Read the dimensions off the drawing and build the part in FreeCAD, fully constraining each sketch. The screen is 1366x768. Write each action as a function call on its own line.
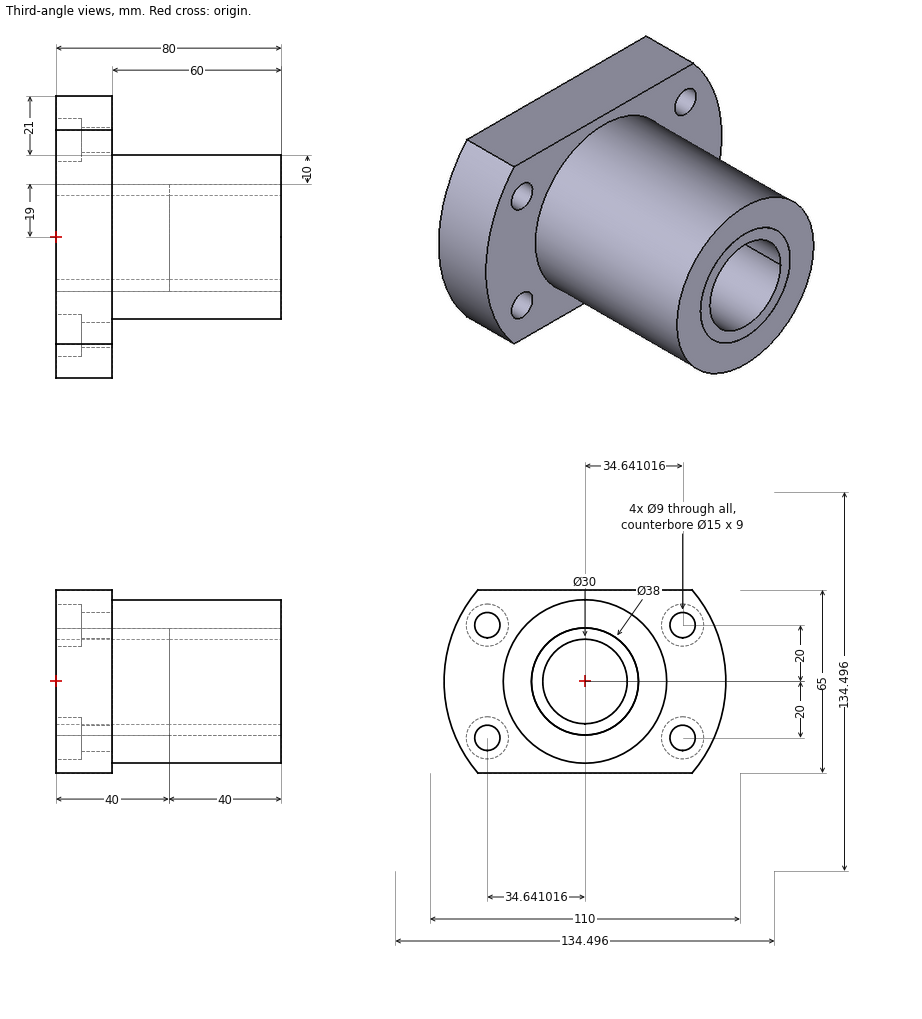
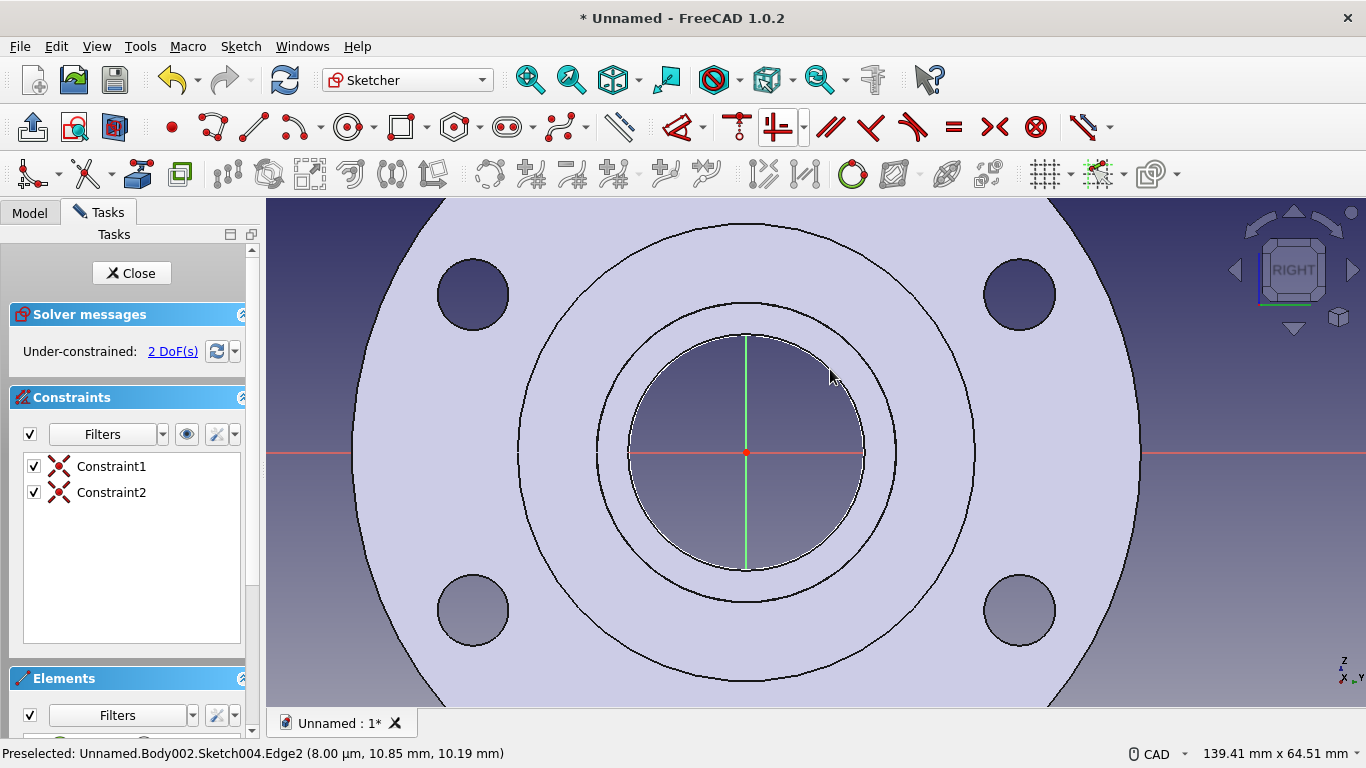
key(d)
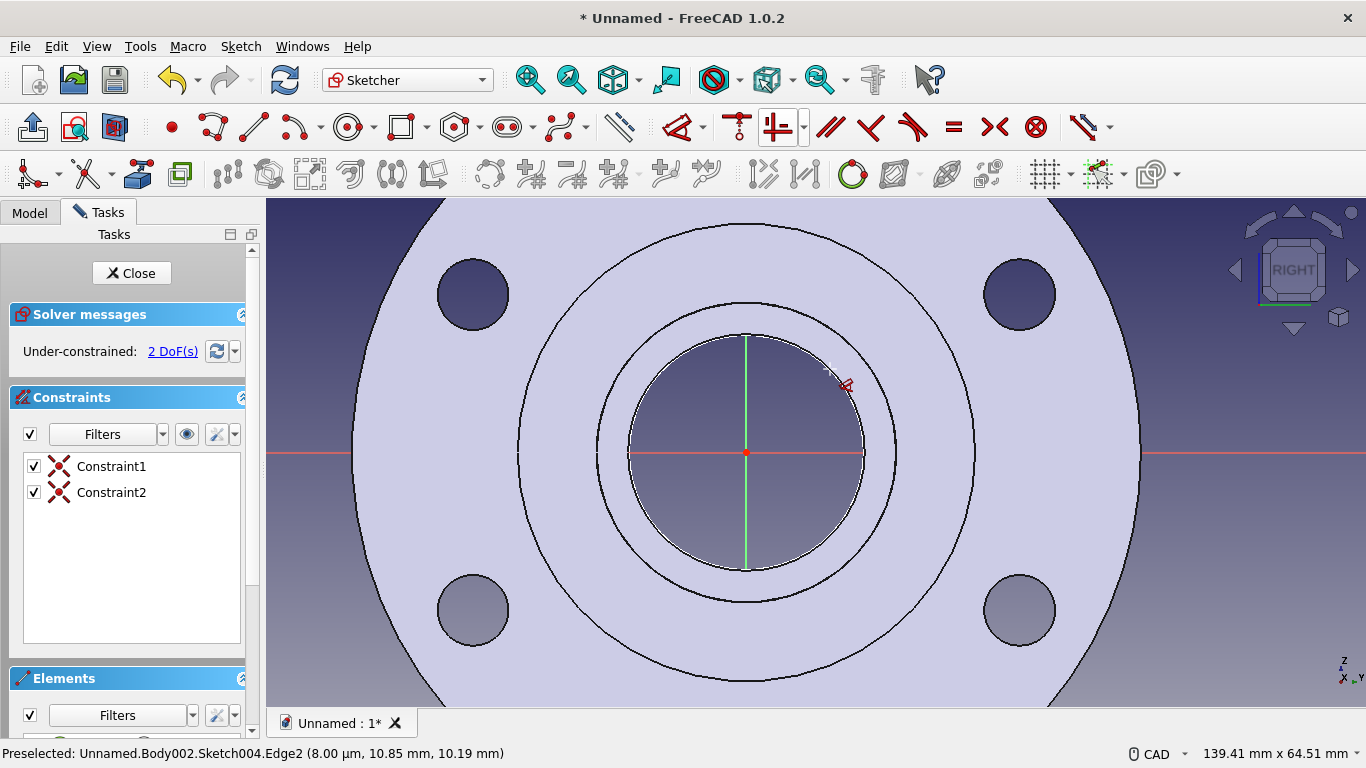
click(852, 347)
click(875, 324)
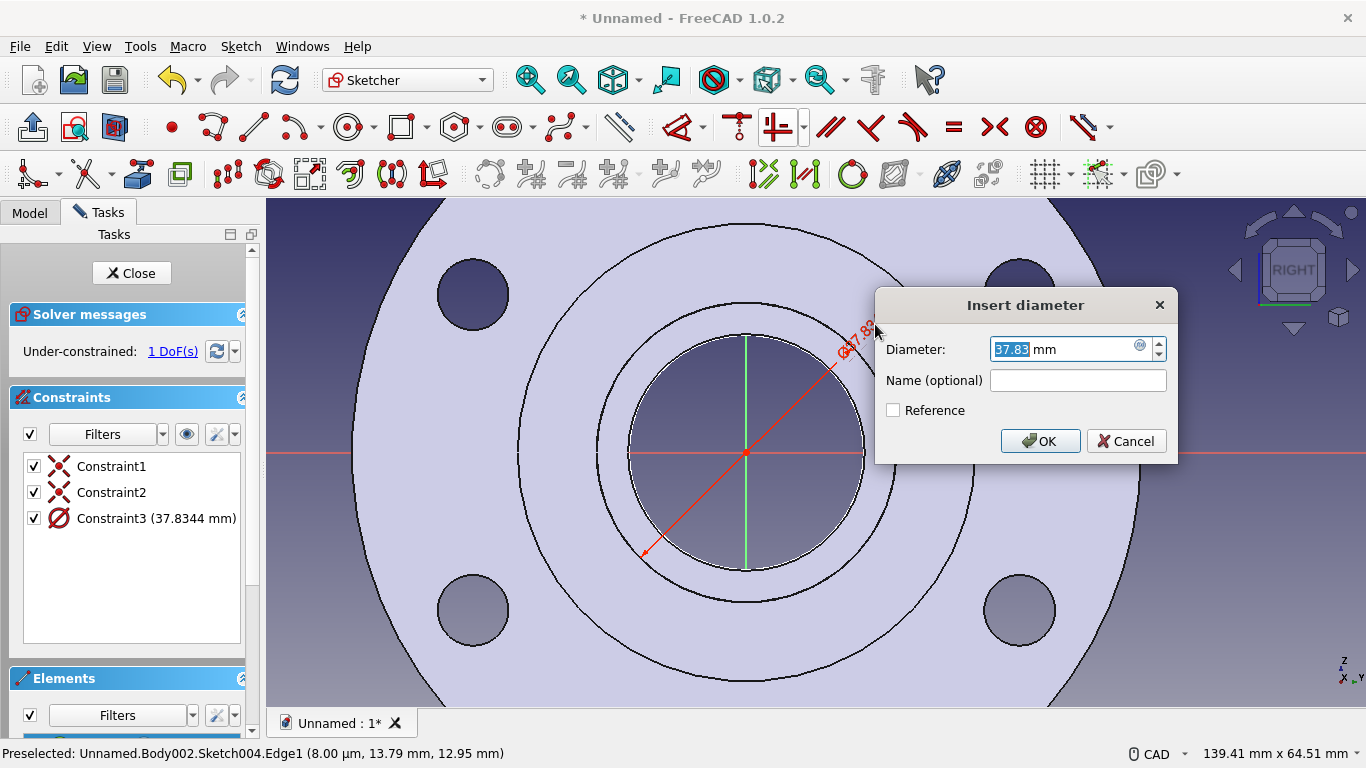
text(38)
key(Return)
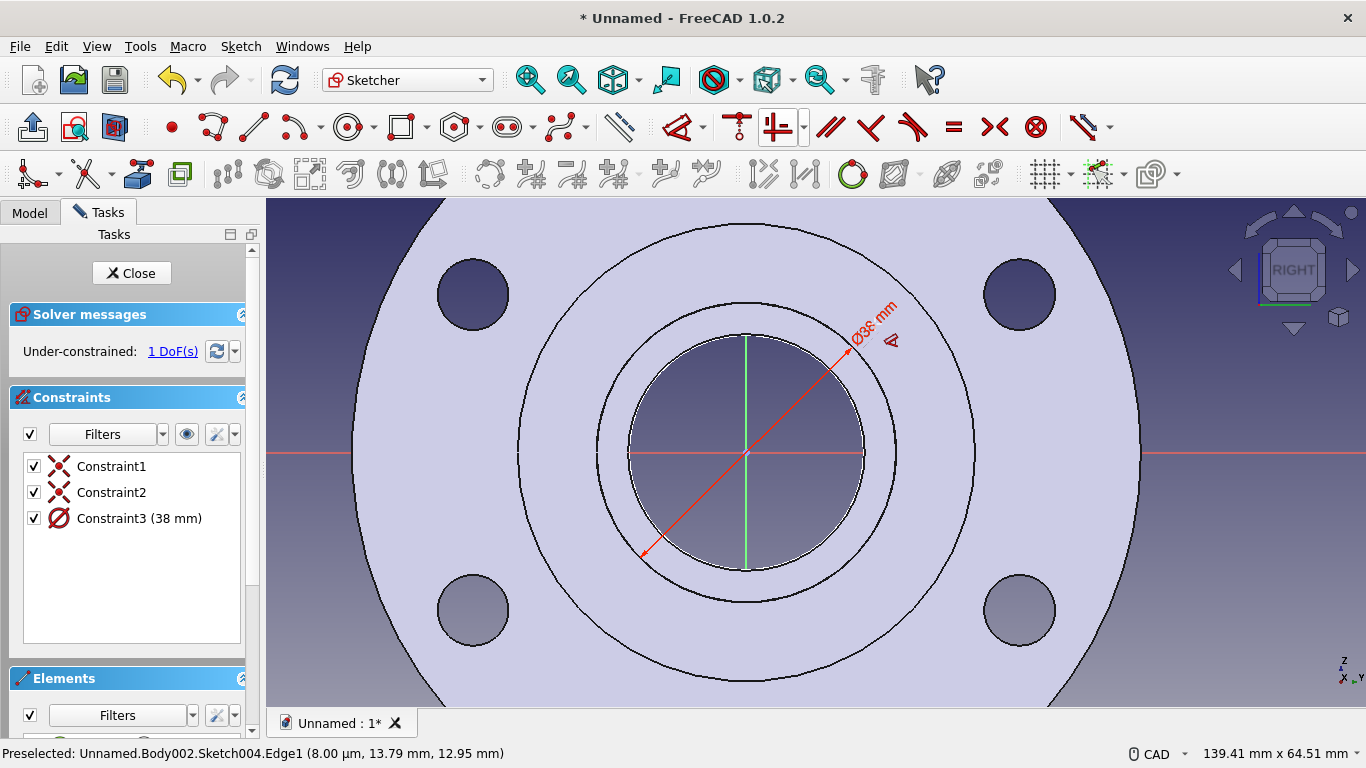
click(829, 369)
click(912, 403)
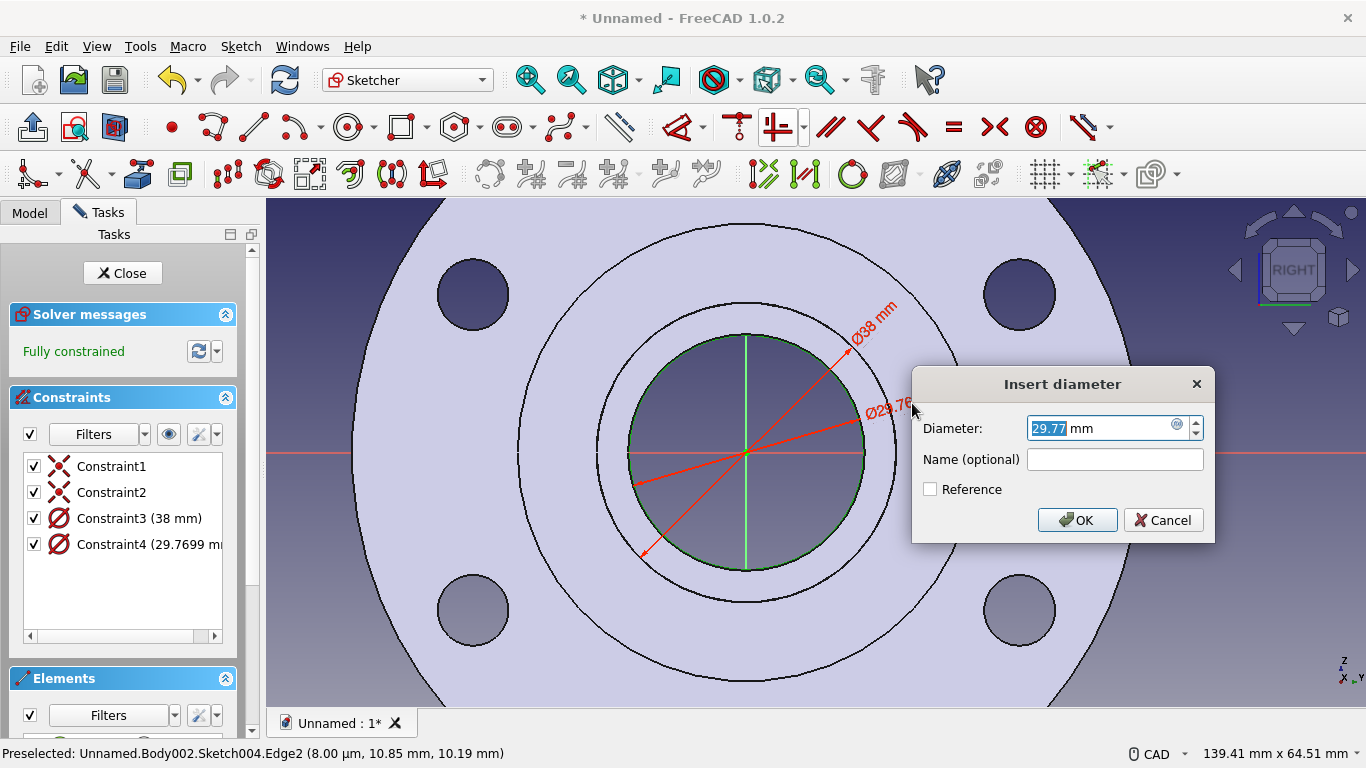
text(30)
key(Return)
key(Escape)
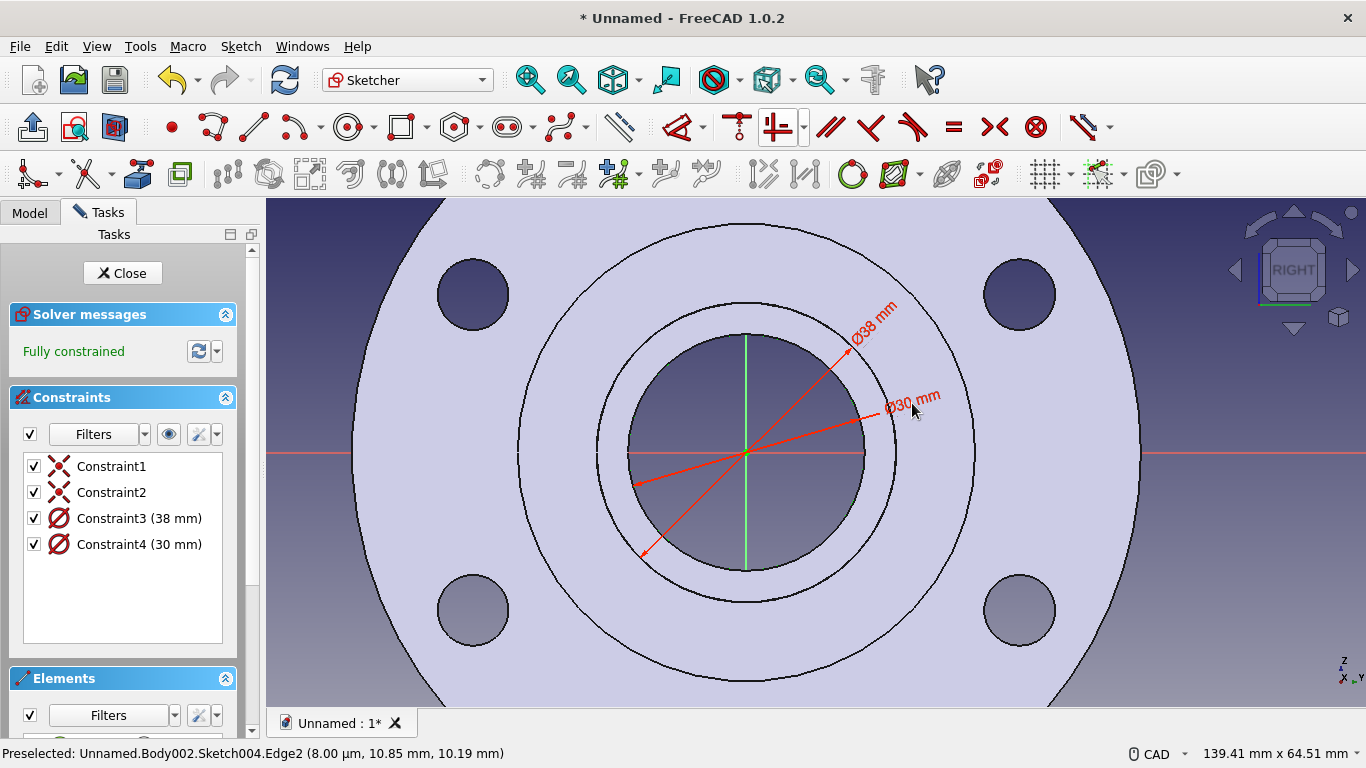
click(123, 273)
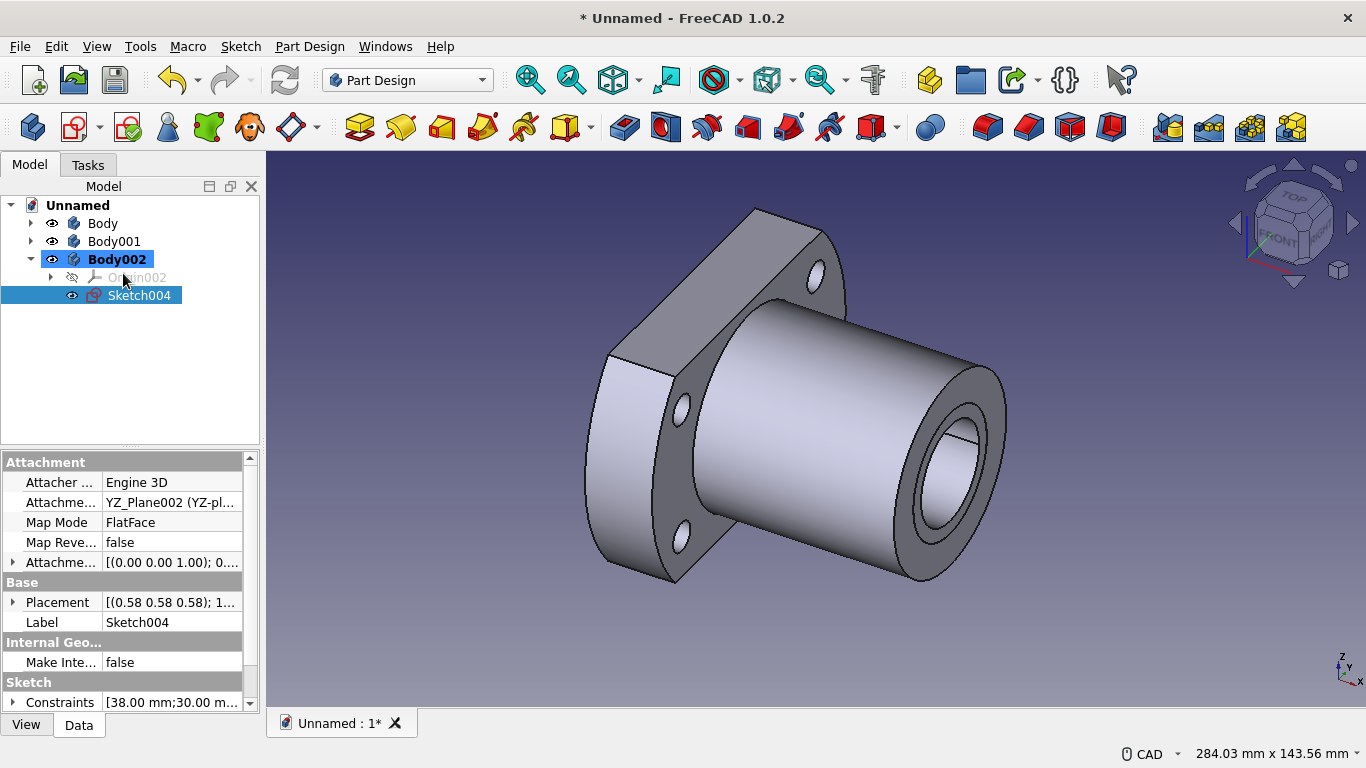
click(360, 128)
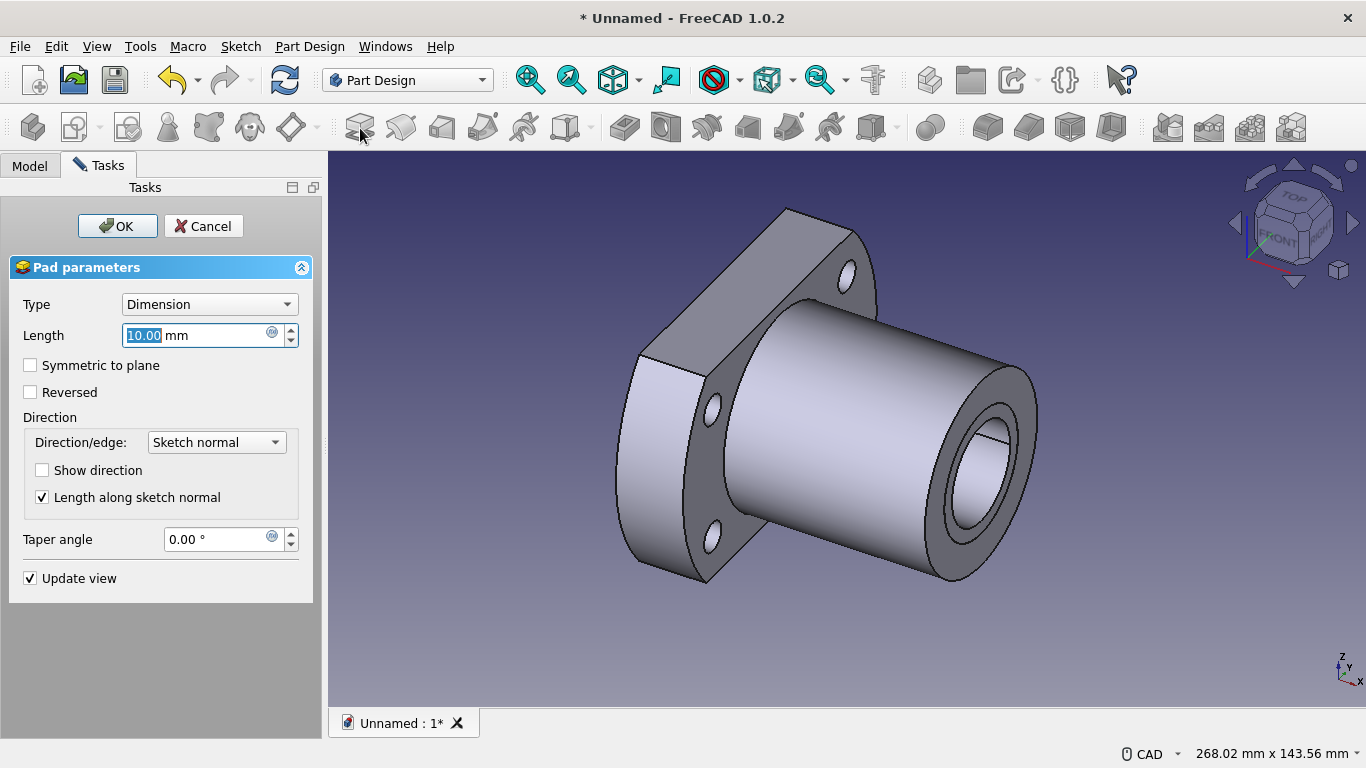
text(40)
key(Tab)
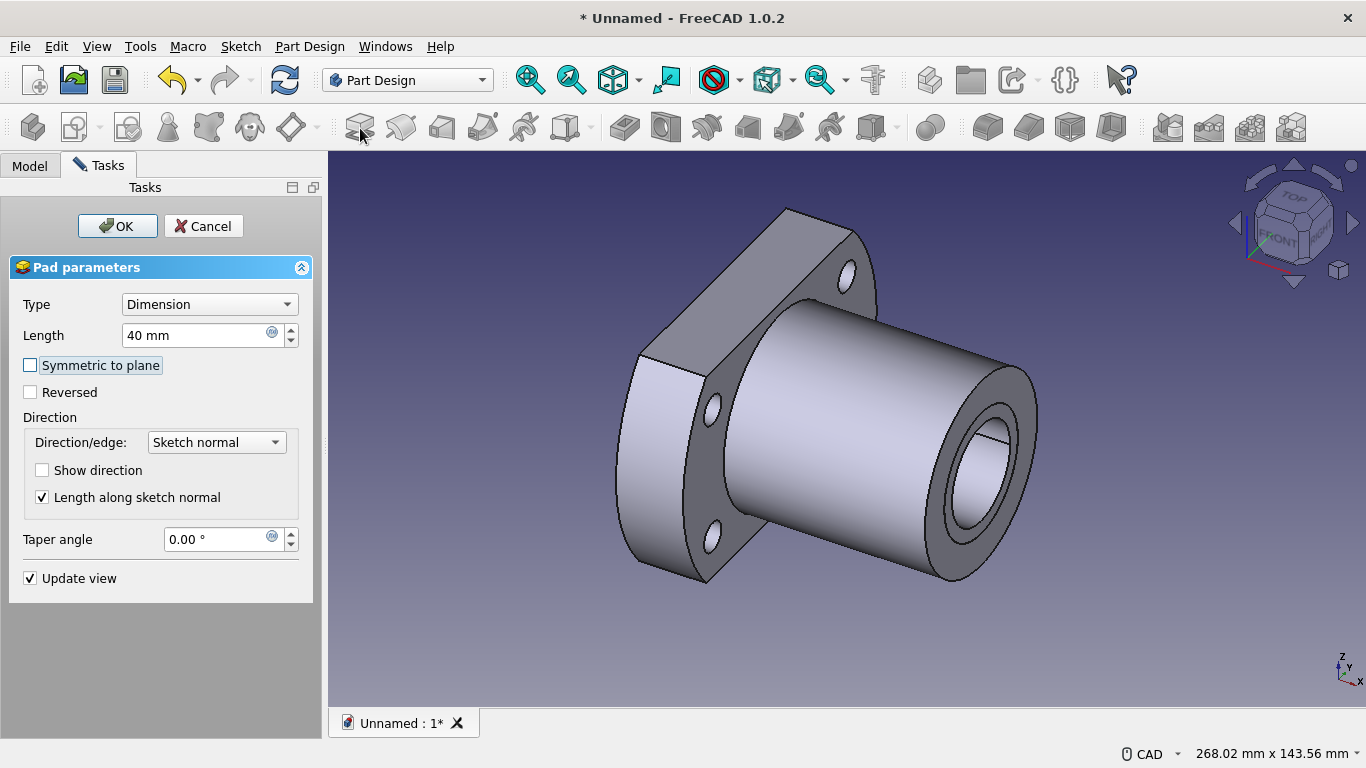
click(118, 226)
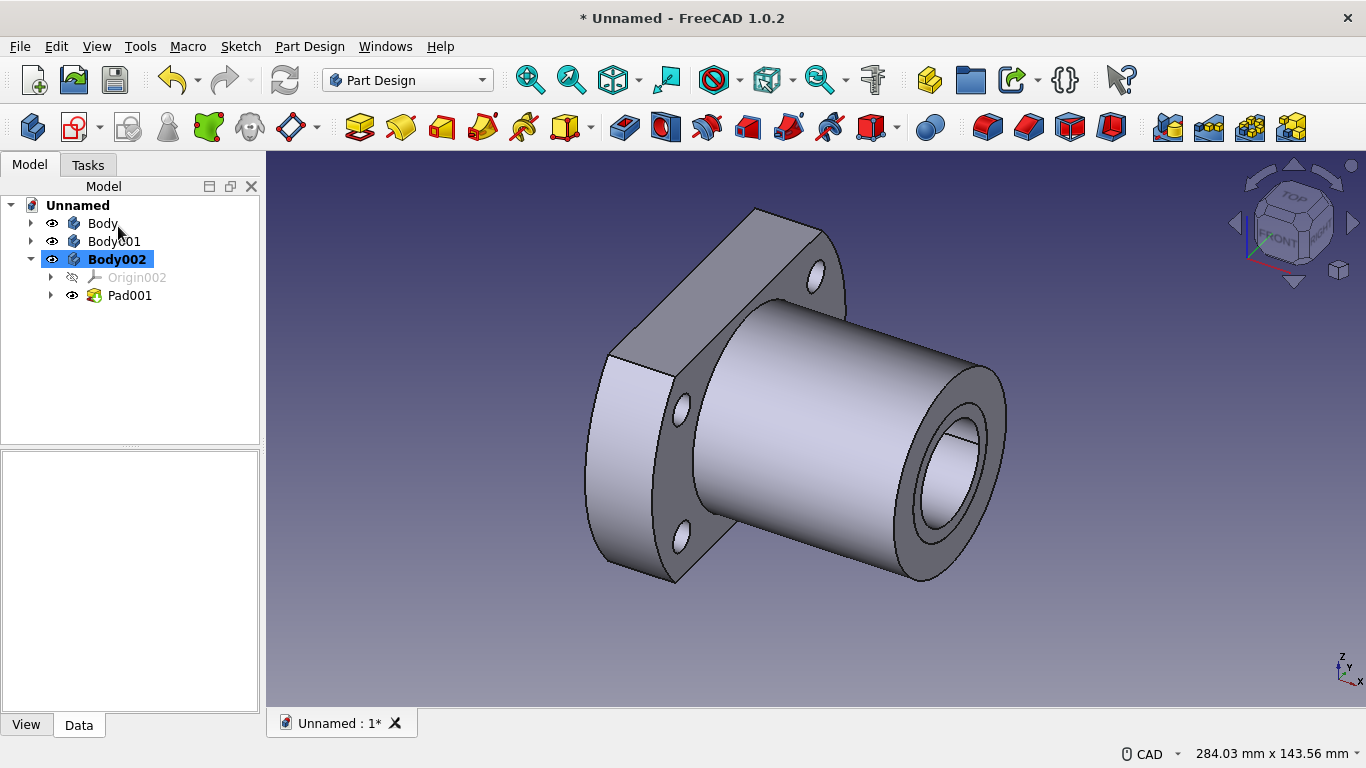
key(0)